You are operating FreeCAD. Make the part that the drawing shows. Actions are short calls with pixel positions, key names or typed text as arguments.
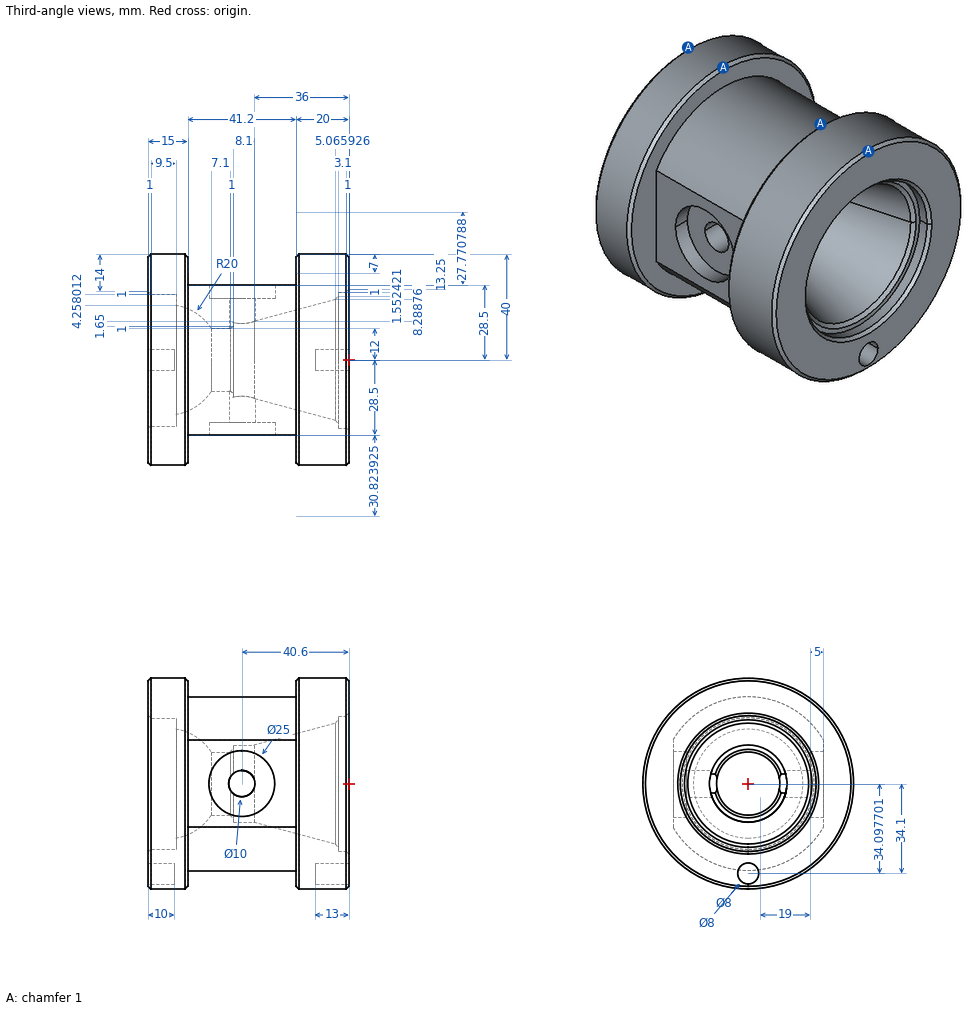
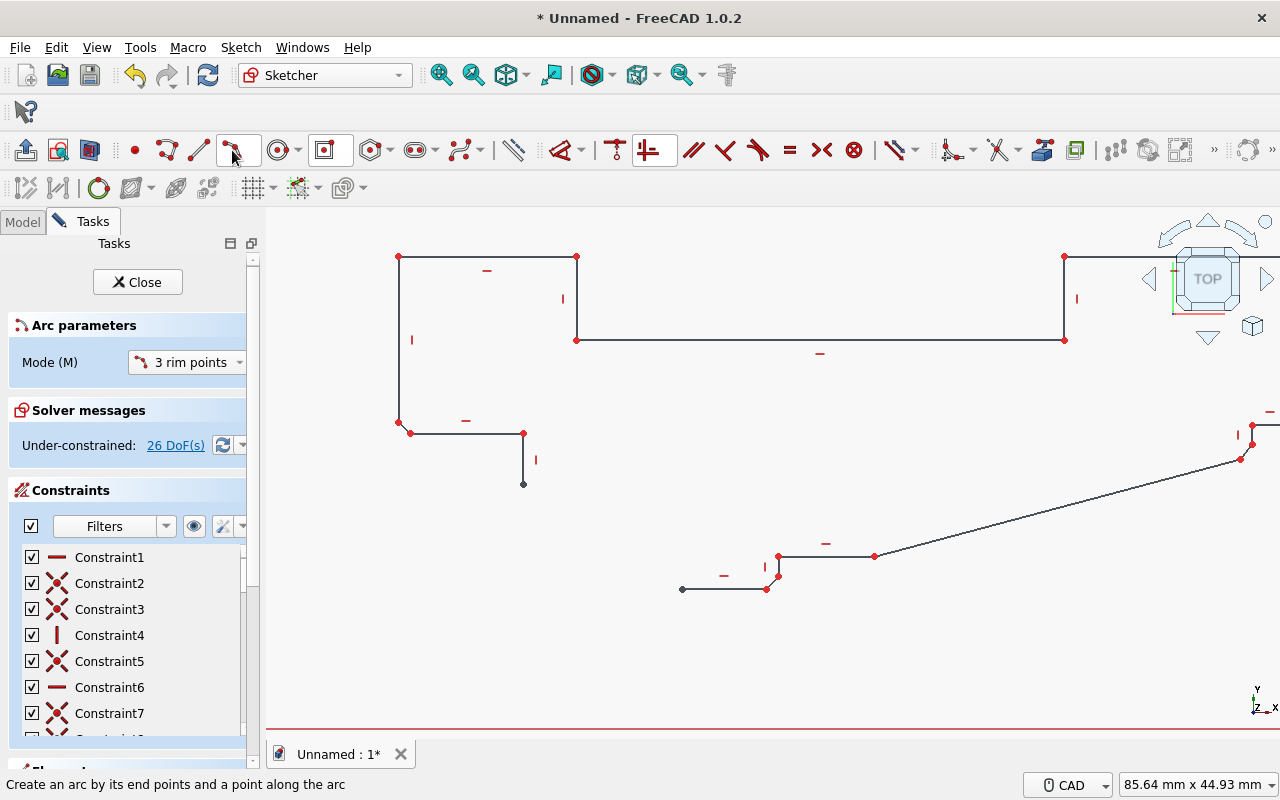
click(523, 485)
click(683, 589)
click(614, 519)
key(Escape)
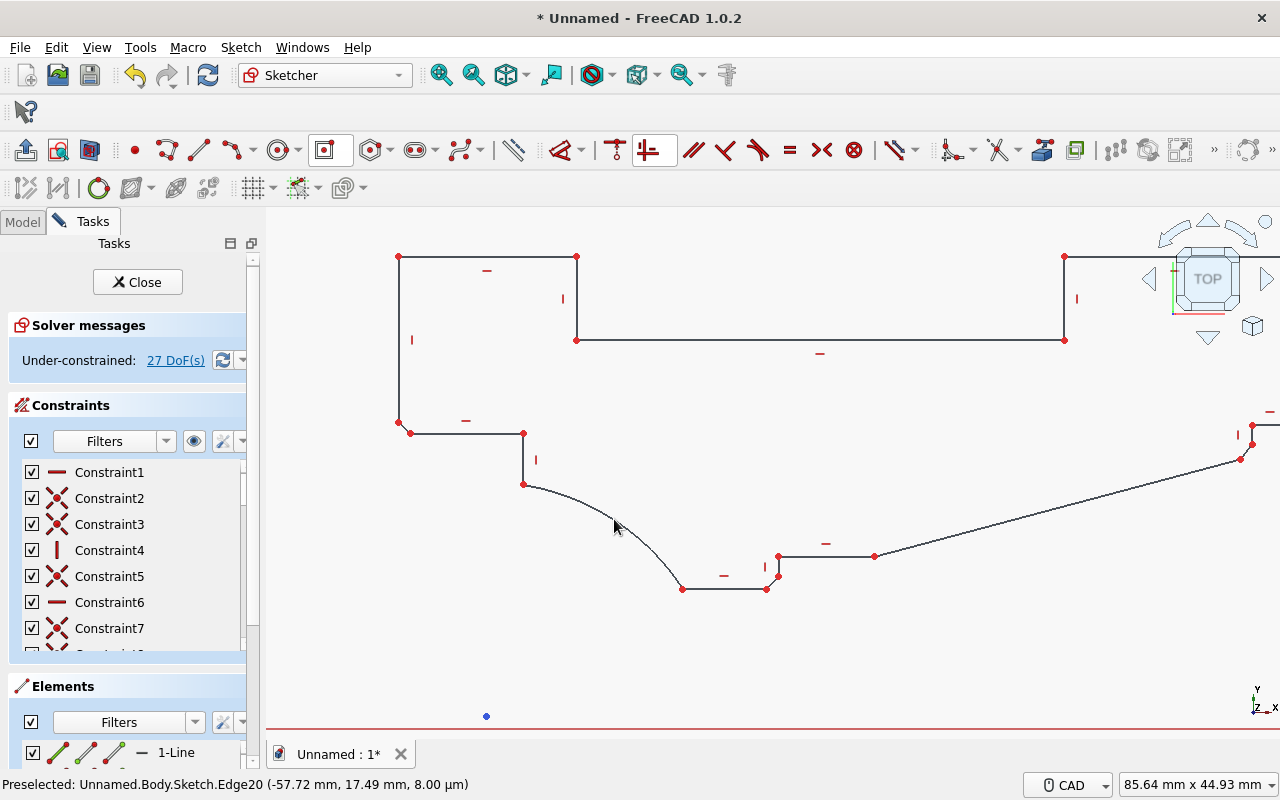
scroll(410, 433, down, 2)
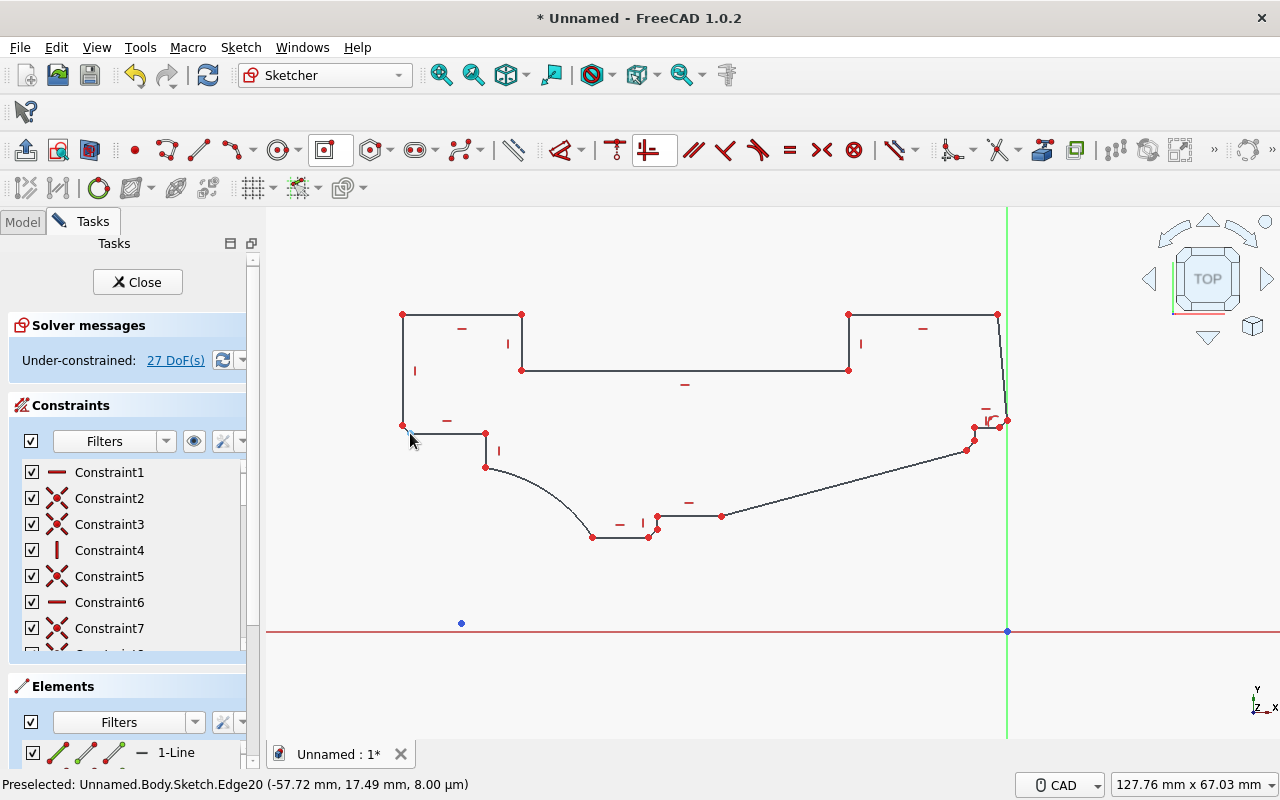
scroll(1000, 347, up, 4)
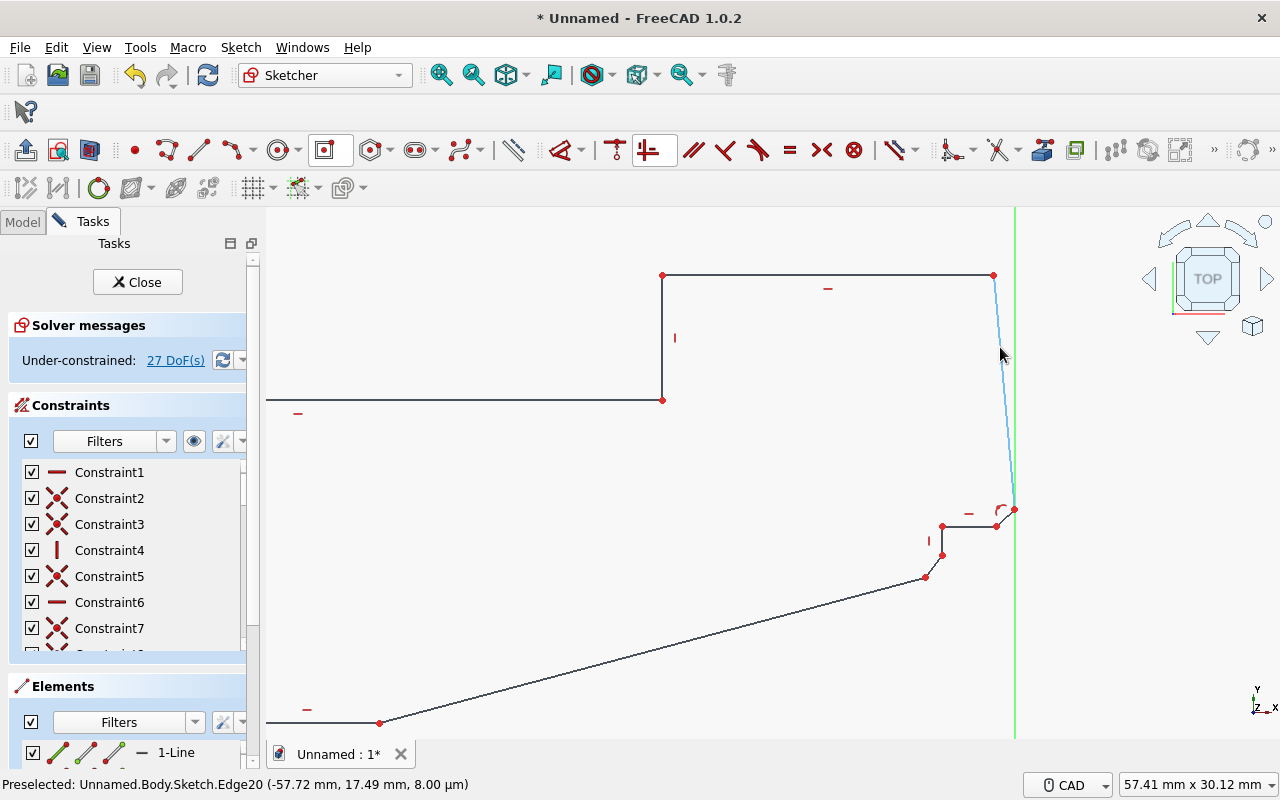
click(1000, 346)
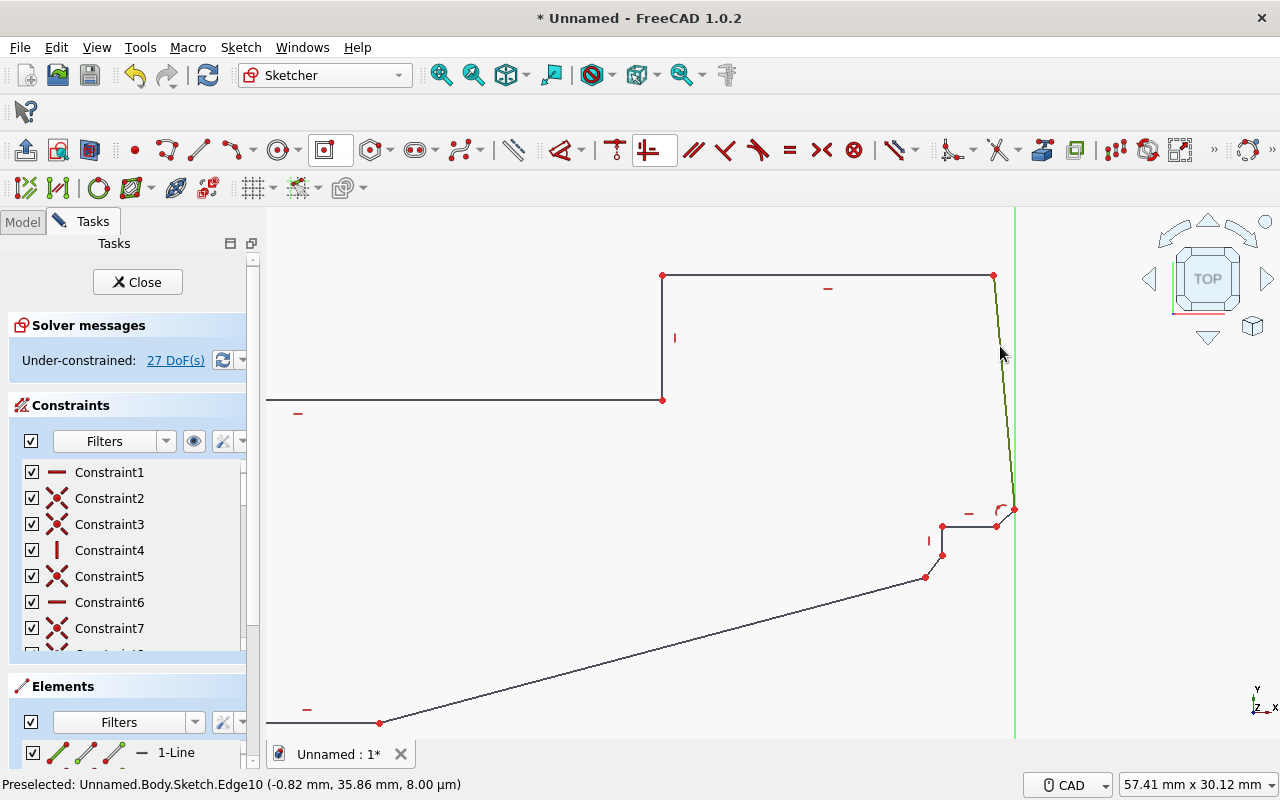
key(v)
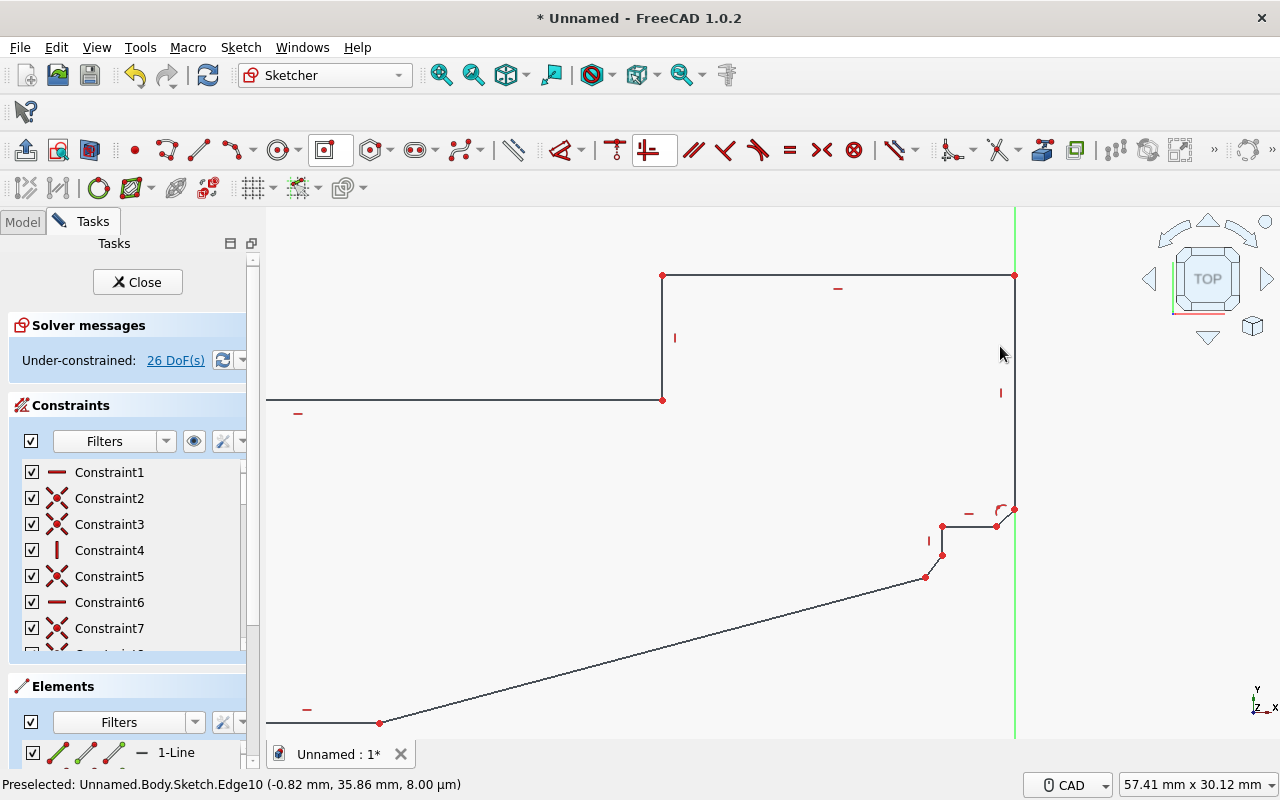
click(560, 150)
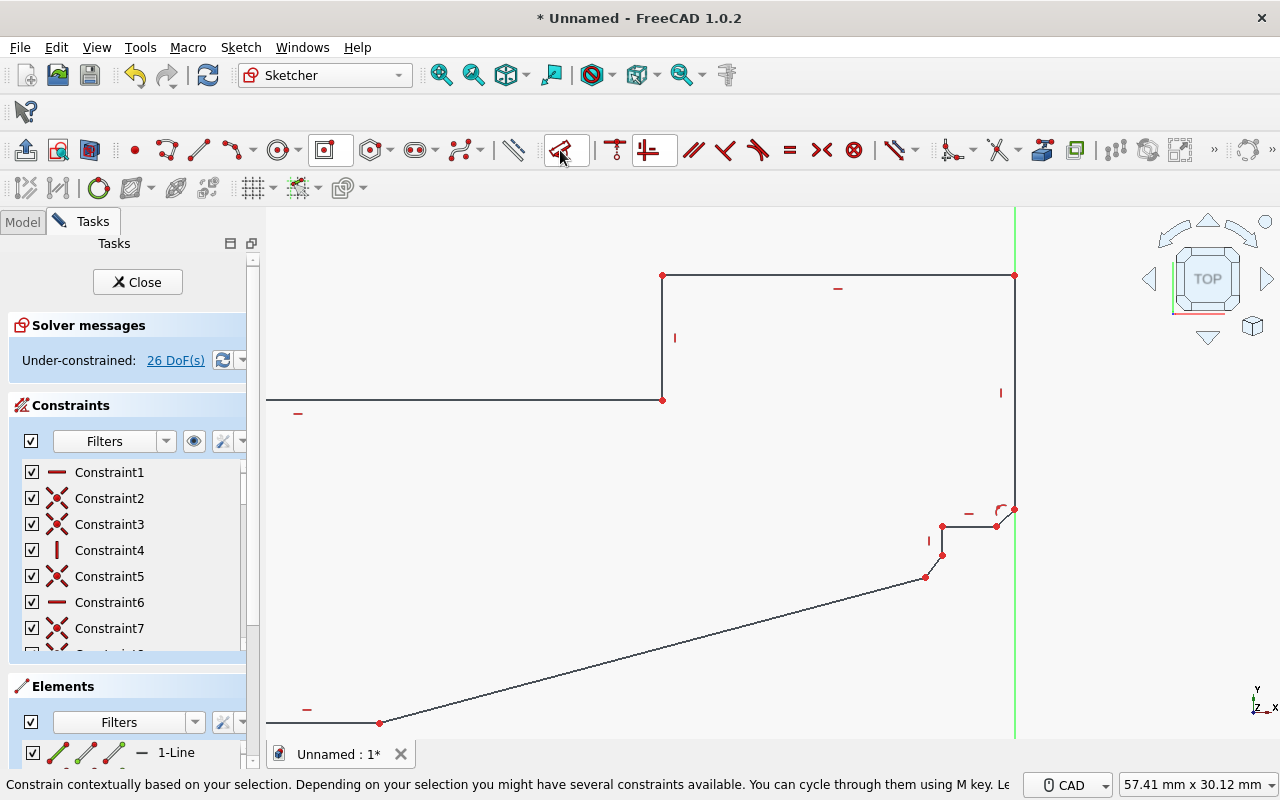
scroll(1000, 347, down, 4)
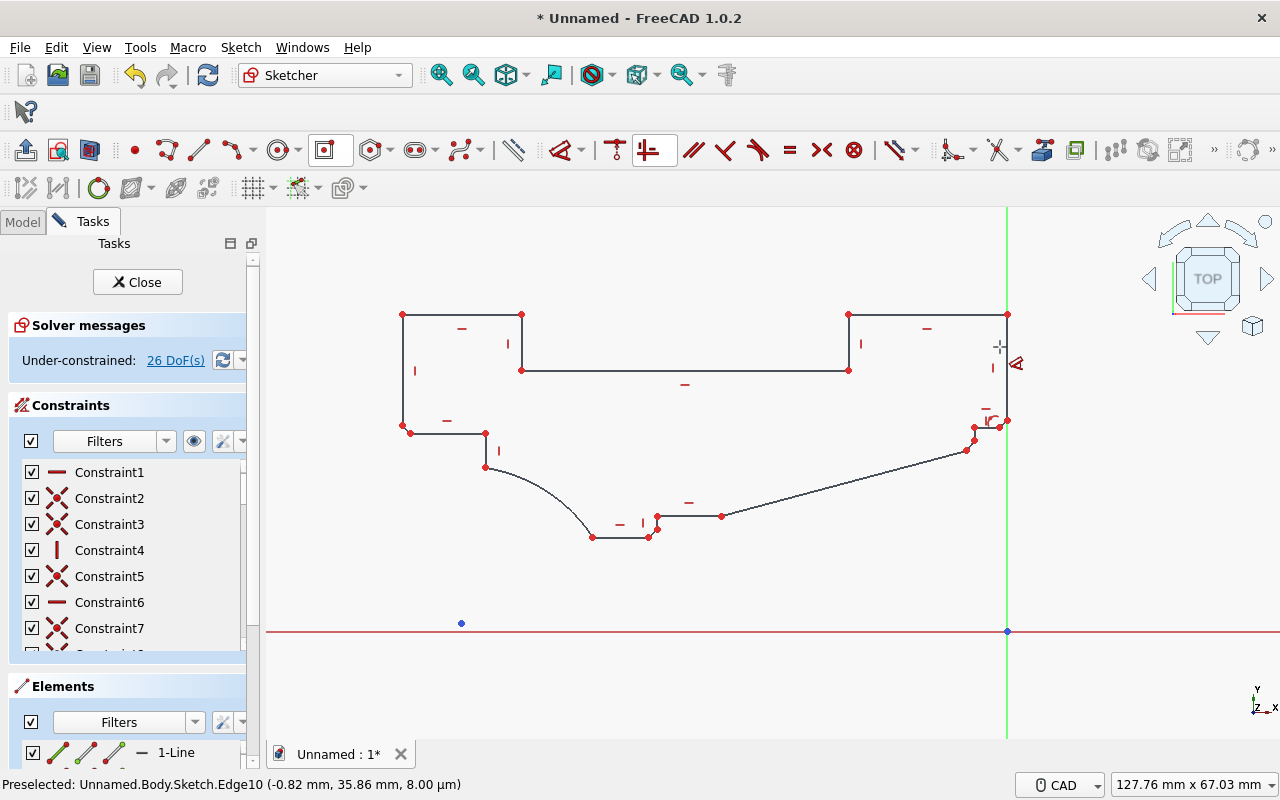
click(568, 508)
click(590, 485)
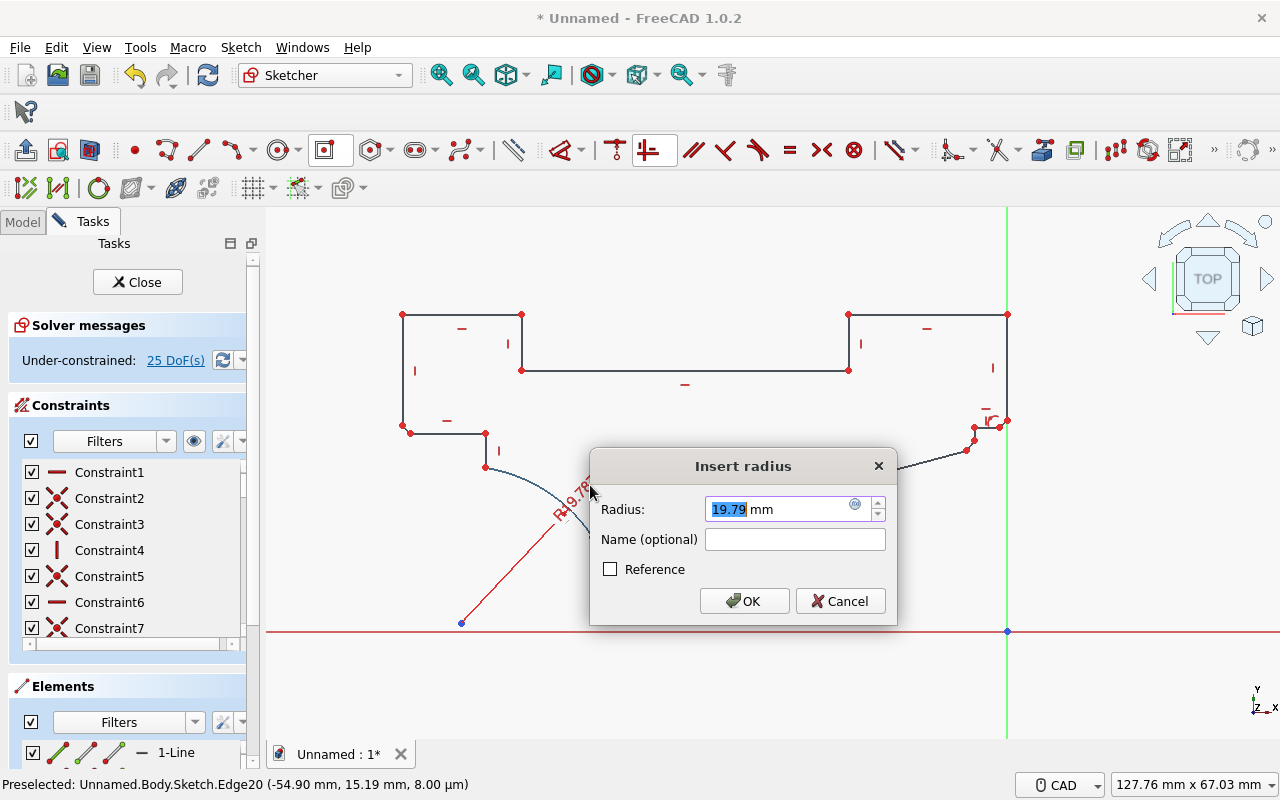
text(20)
key(Return)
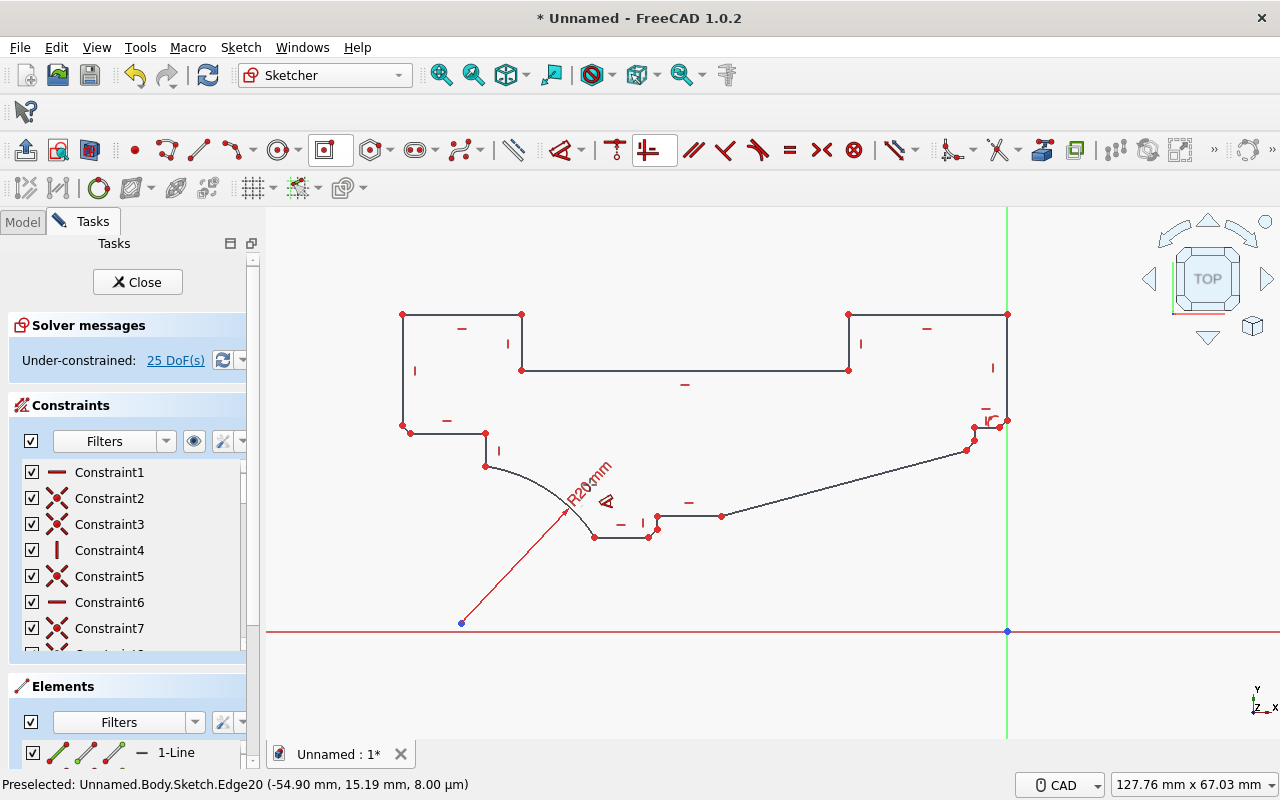
click(849, 332)
click(883, 343)